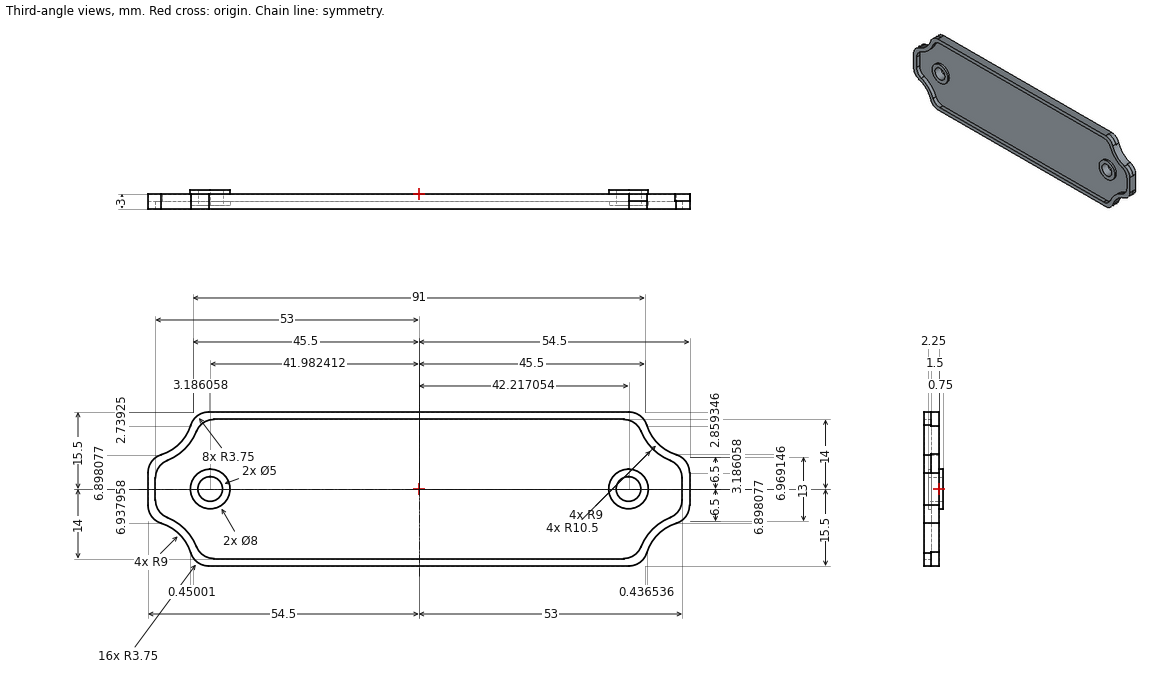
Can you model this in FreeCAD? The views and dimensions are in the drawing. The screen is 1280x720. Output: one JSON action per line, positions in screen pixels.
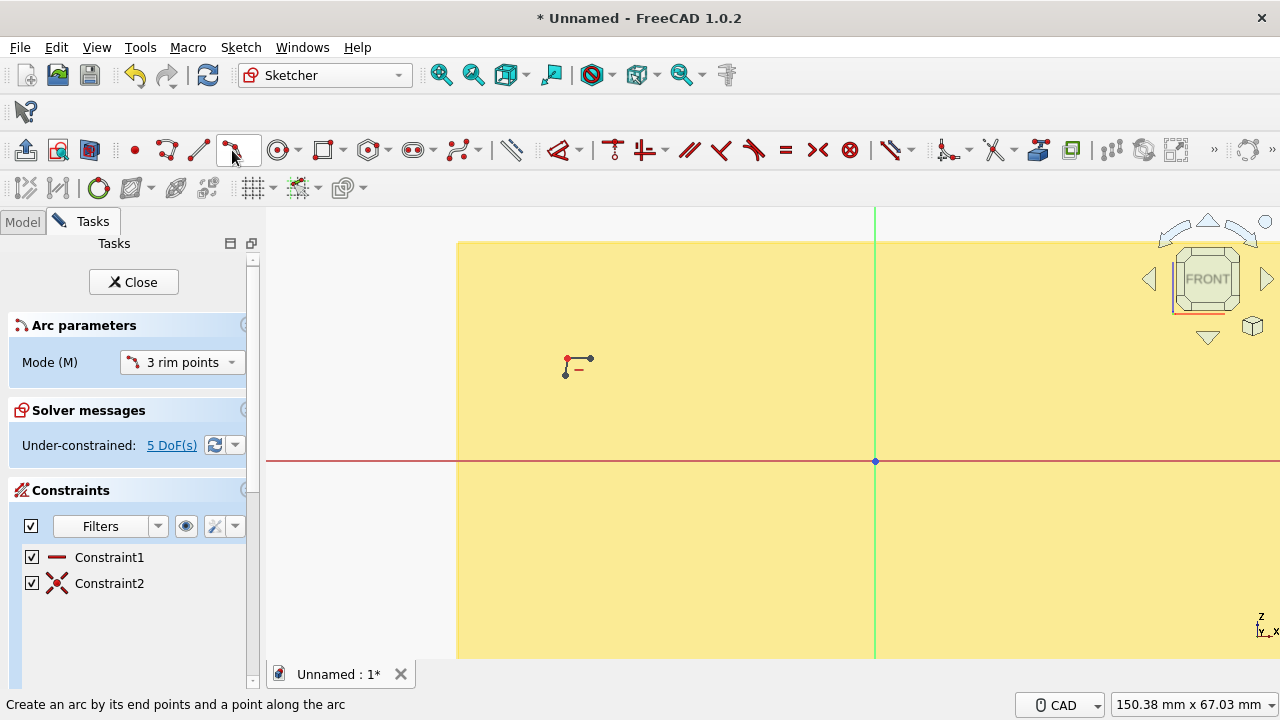
{"action": "scroll", "coordinate": [565, 375], "scroll_direction": "up", "scroll_amount": 3}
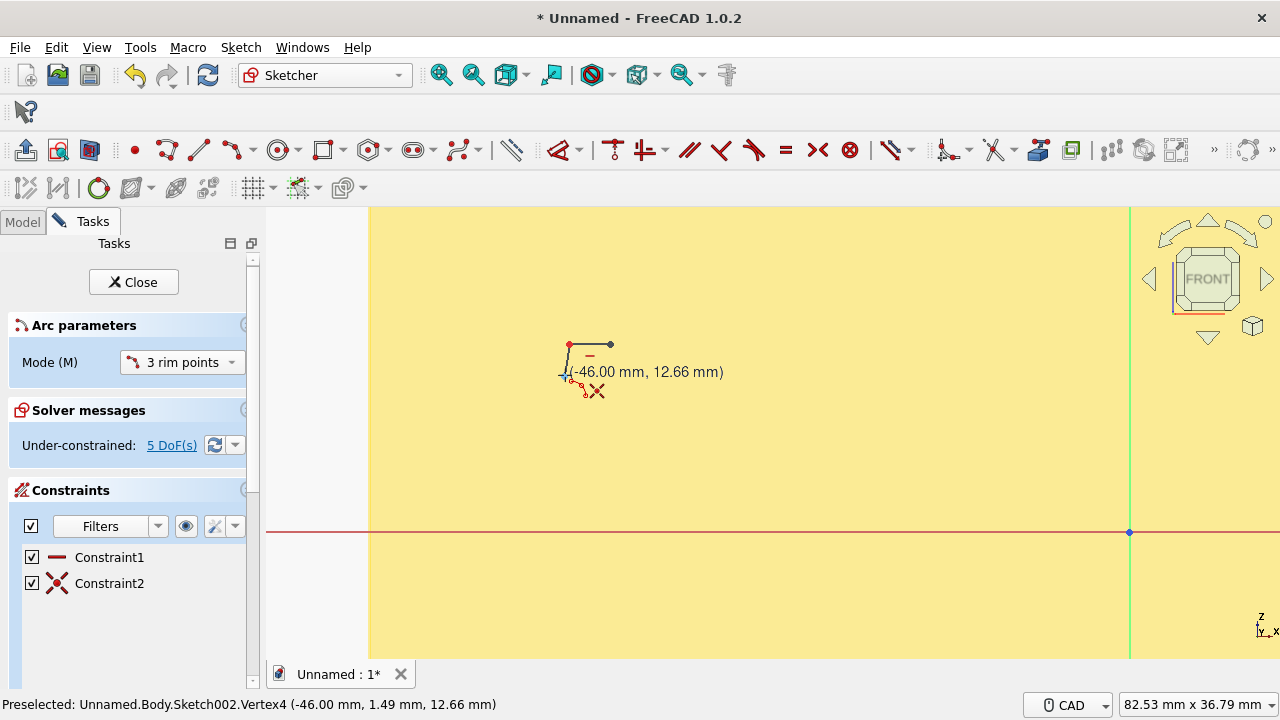
{"action": "left_click", "coordinate": [565, 377]}
{"action": "left_click", "coordinate": [611, 344]}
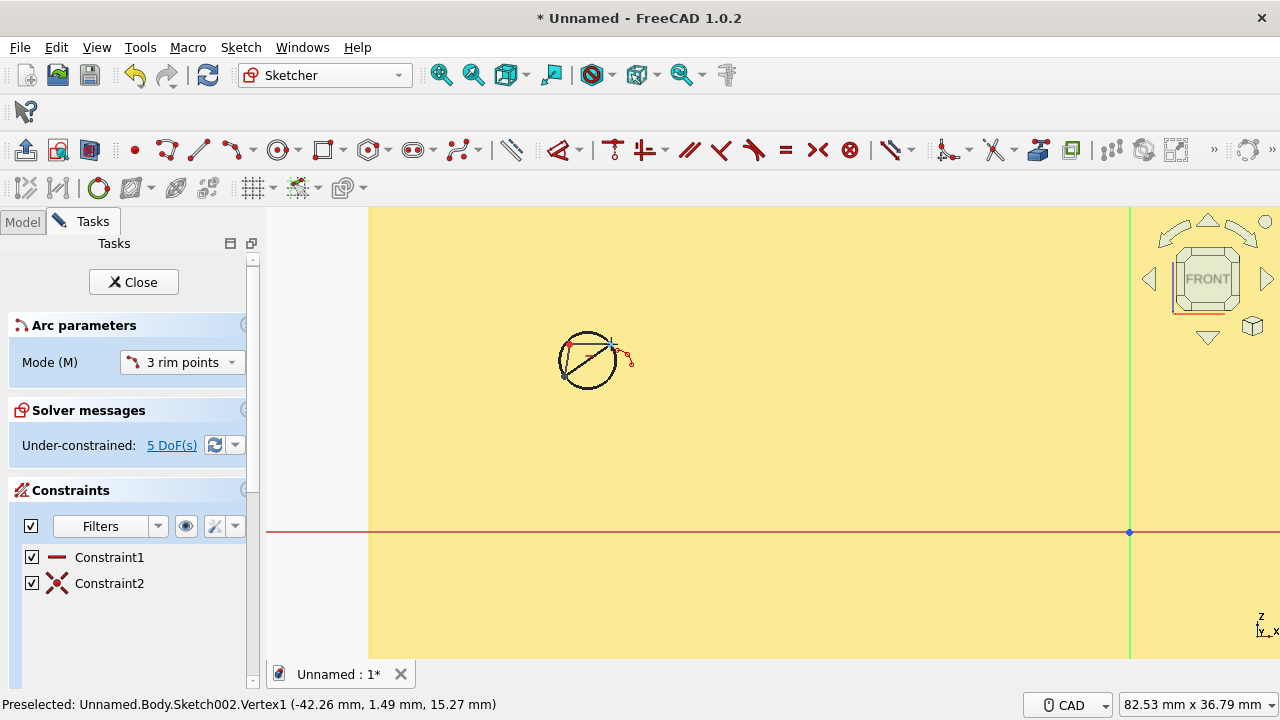
{"action": "scroll", "coordinate": [582, 351], "scroll_direction": "up", "scroll_amount": 3}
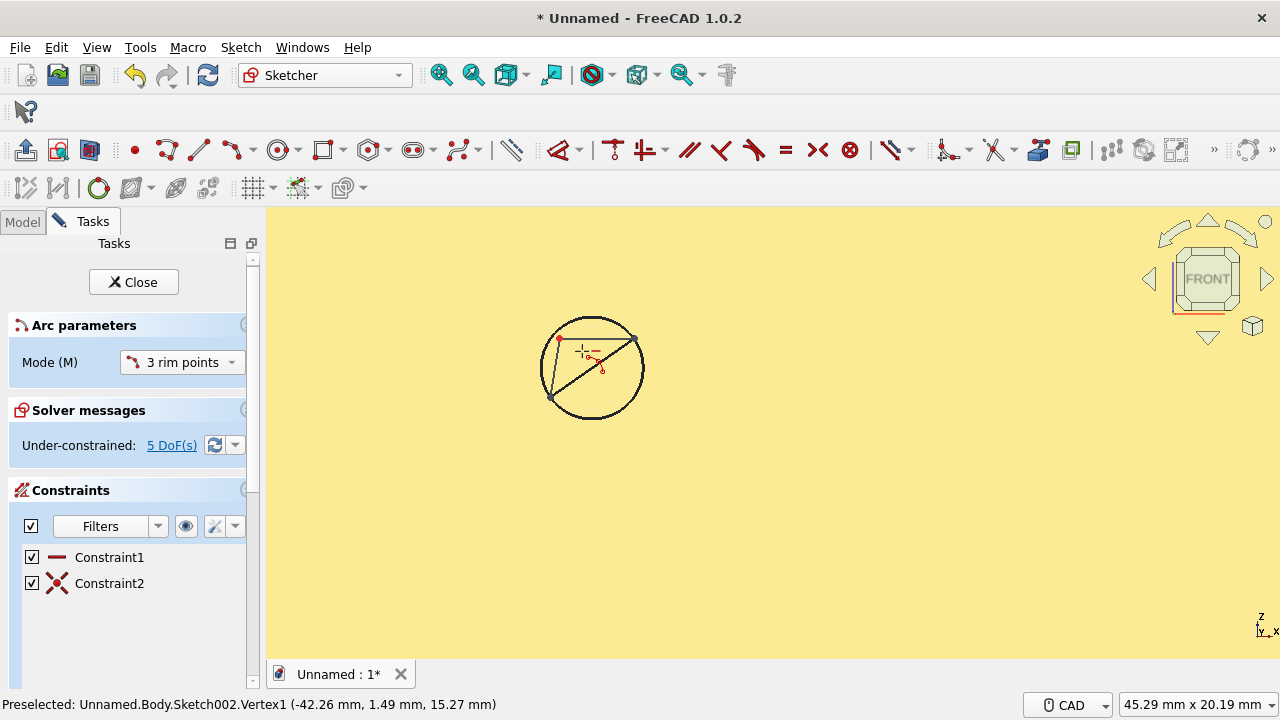
{"action": "left_click", "coordinate": [582, 351]}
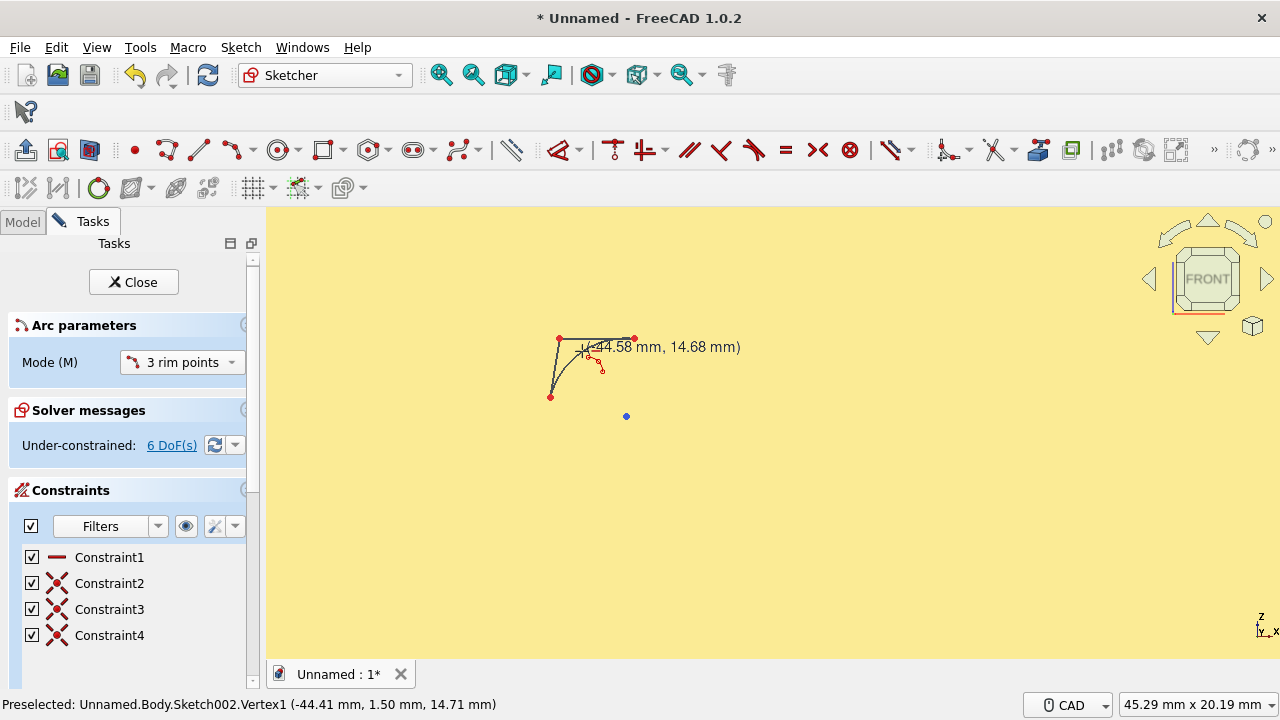
{"action": "left_click", "coordinate": [168, 150]}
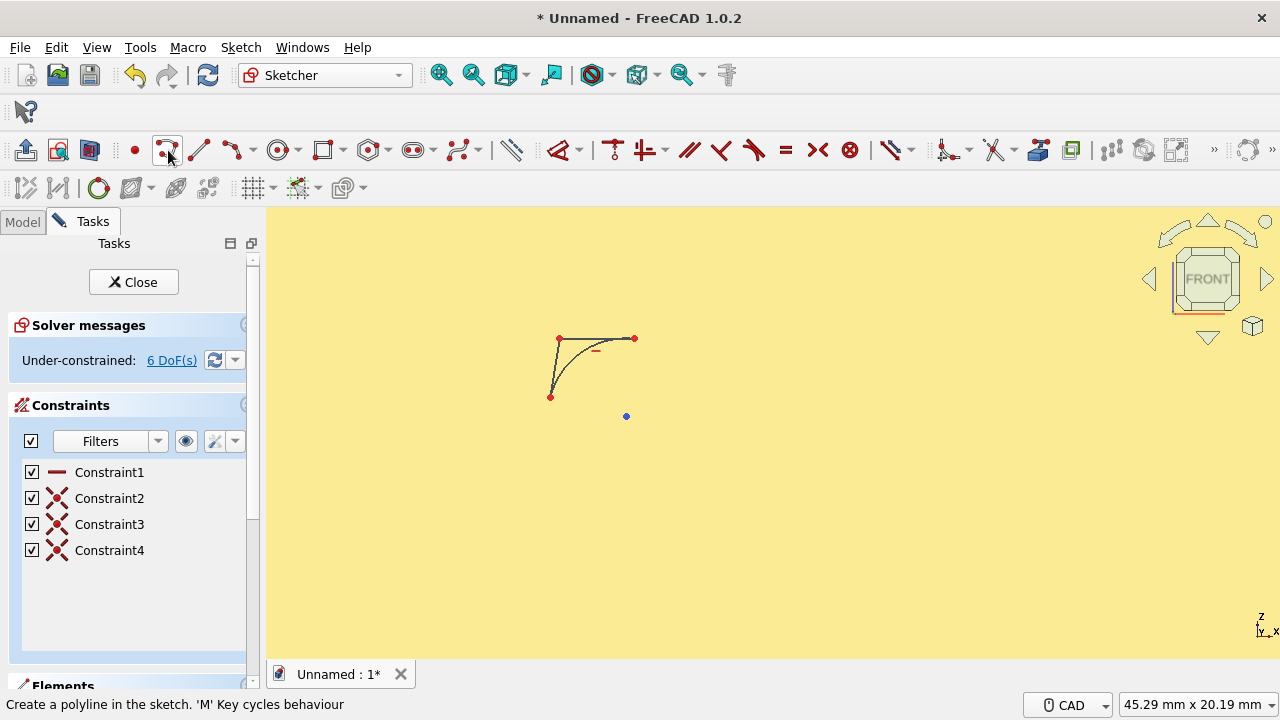
{"action": "scroll", "coordinate": [418, 352], "scroll_direction": "down", "scroll_amount": 7}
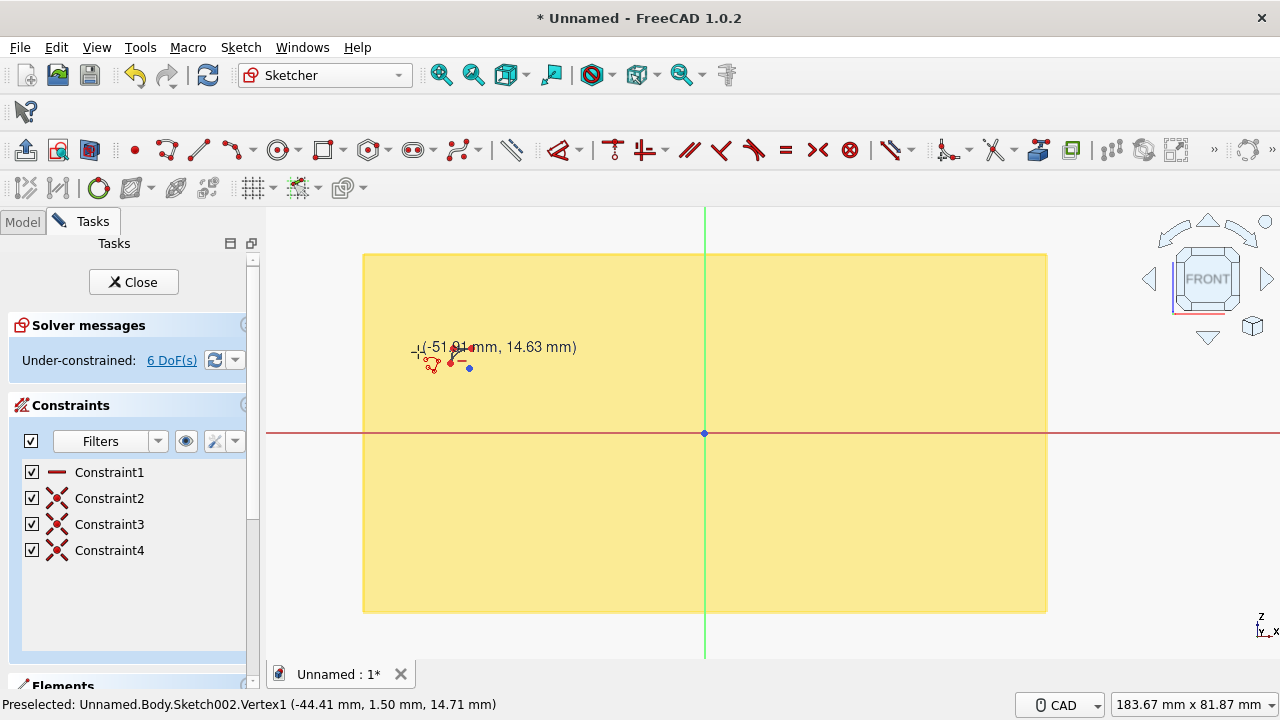
{"action": "left_click", "coordinate": [958, 363]}
{"action": "left_click", "coordinate": [956, 348]}
{"action": "left_click", "coordinate": [938, 348]}
{"action": "right_click", "coordinate": [938, 348]}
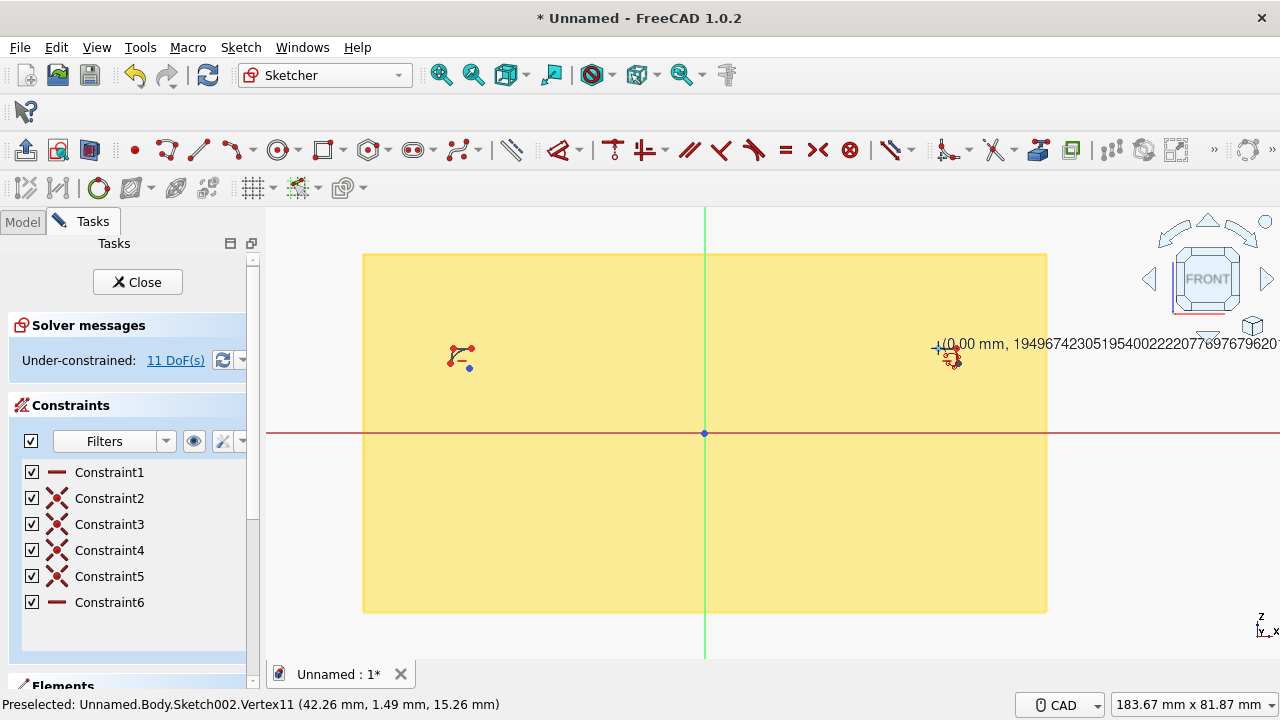
{"action": "left_click", "coordinate": [232, 150]}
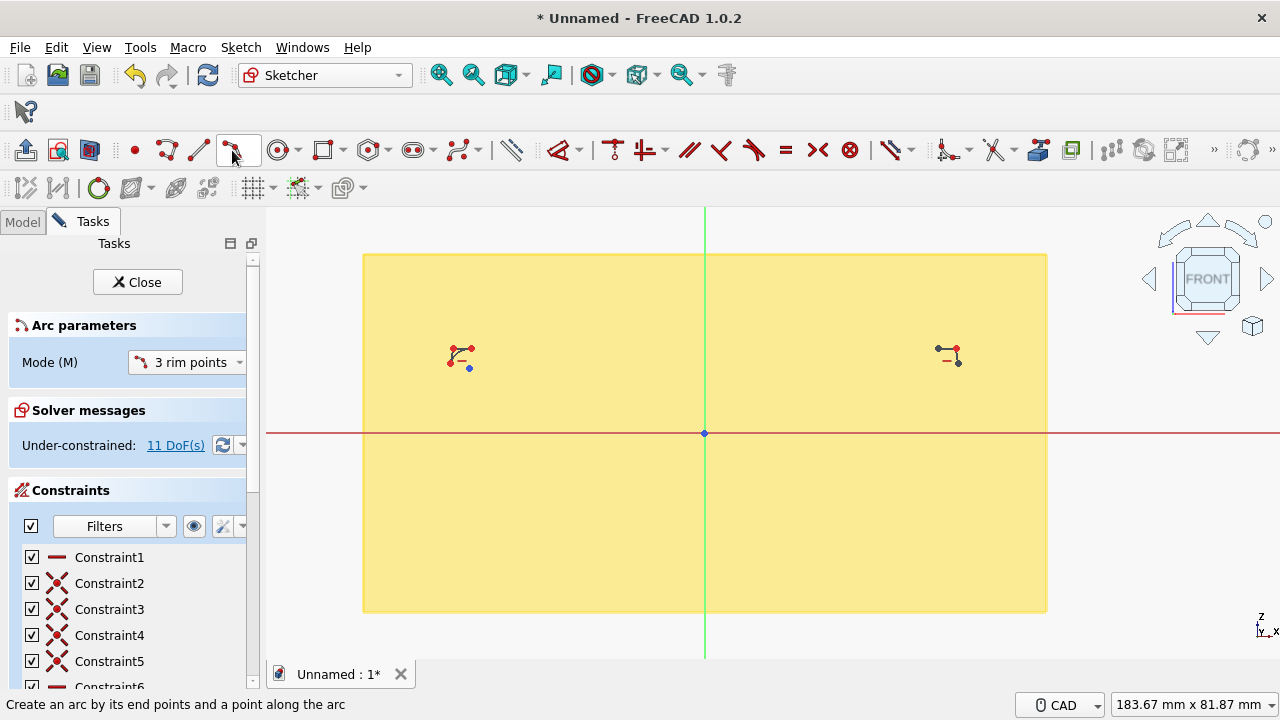
{"action": "scroll", "coordinate": [938, 348], "scroll_direction": "up", "scroll_amount": 3}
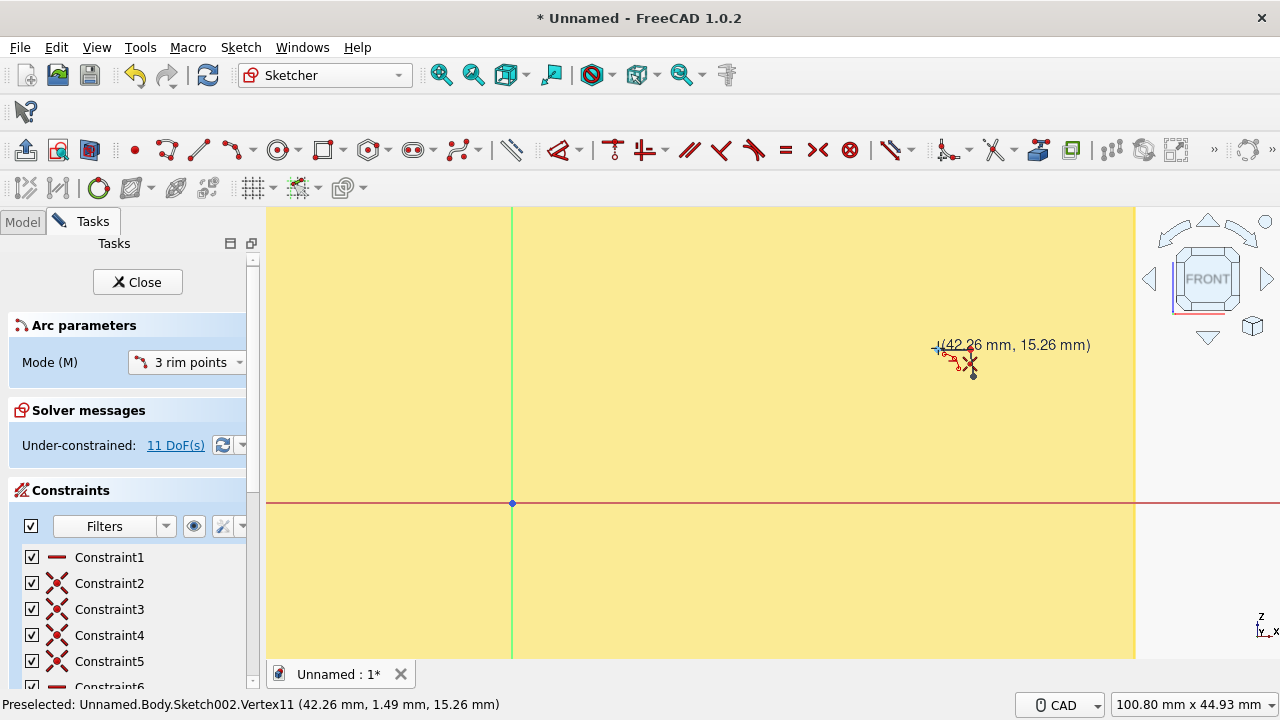
{"action": "left_click", "coordinate": [937, 350]}
{"action": "left_click", "coordinate": [974, 377]}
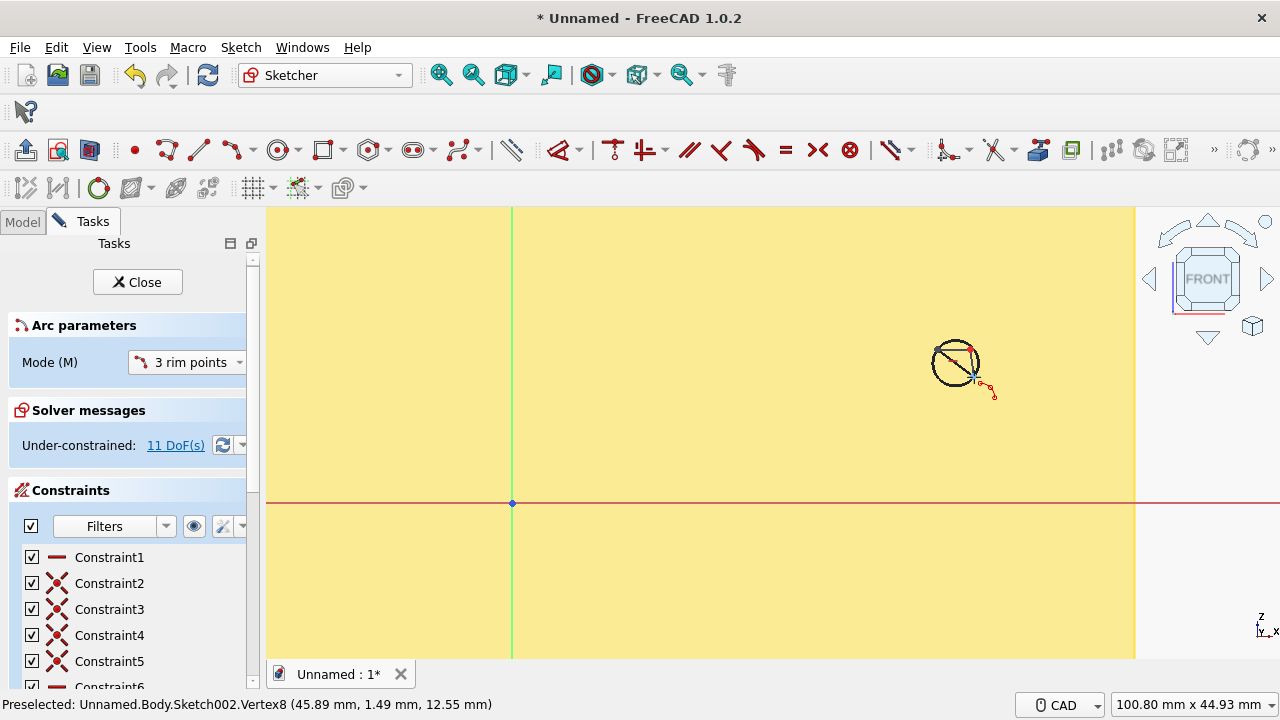
{"action": "scroll", "coordinate": [961, 355], "scroll_direction": "up", "scroll_amount": 4}